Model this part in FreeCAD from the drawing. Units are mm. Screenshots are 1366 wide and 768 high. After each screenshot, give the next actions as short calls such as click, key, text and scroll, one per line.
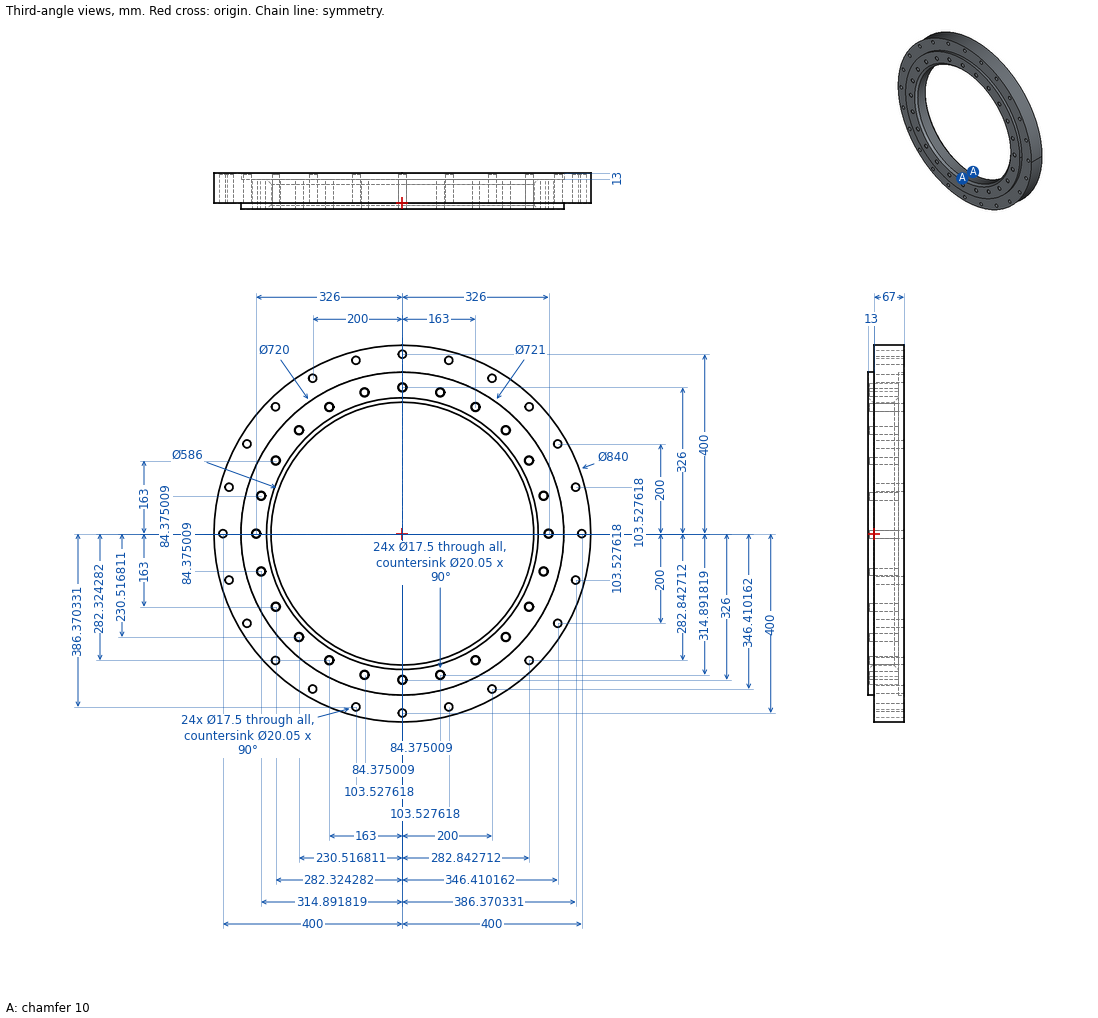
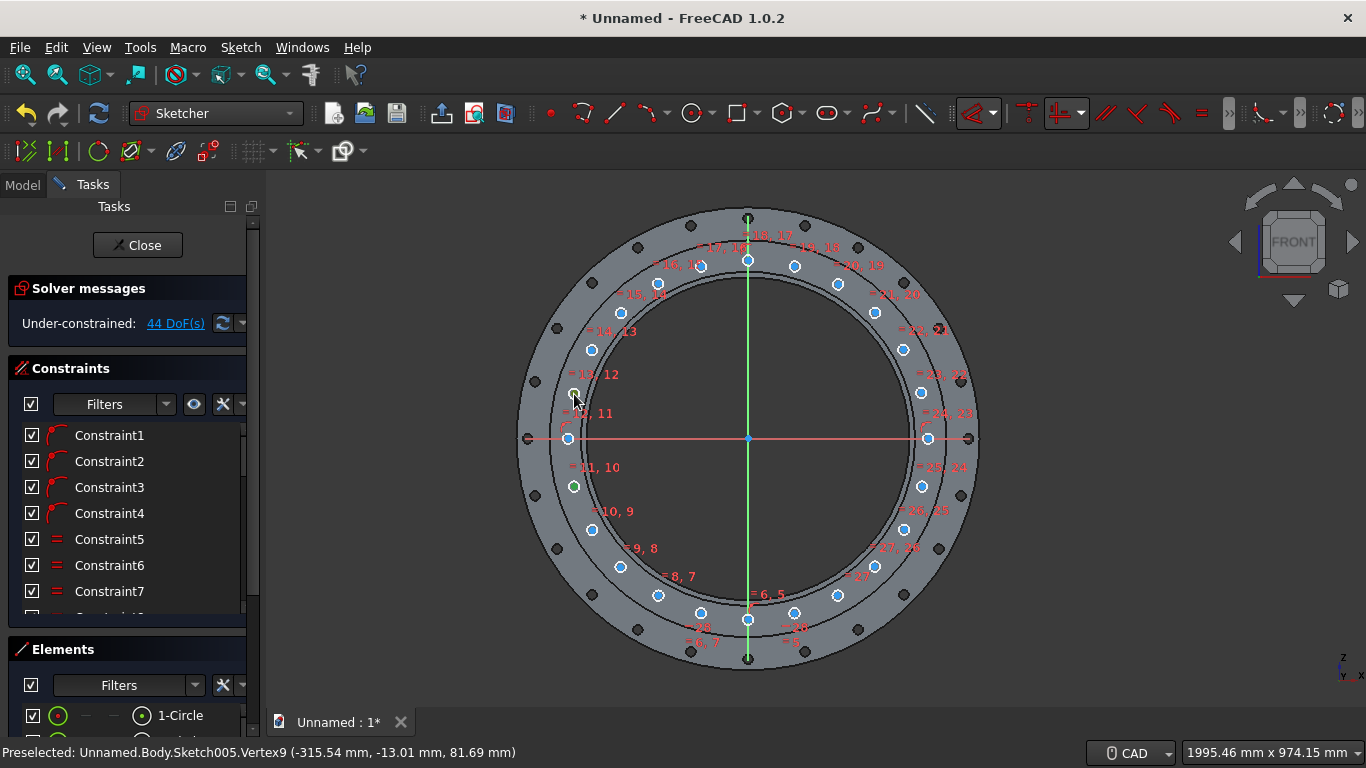
click(1084, 114)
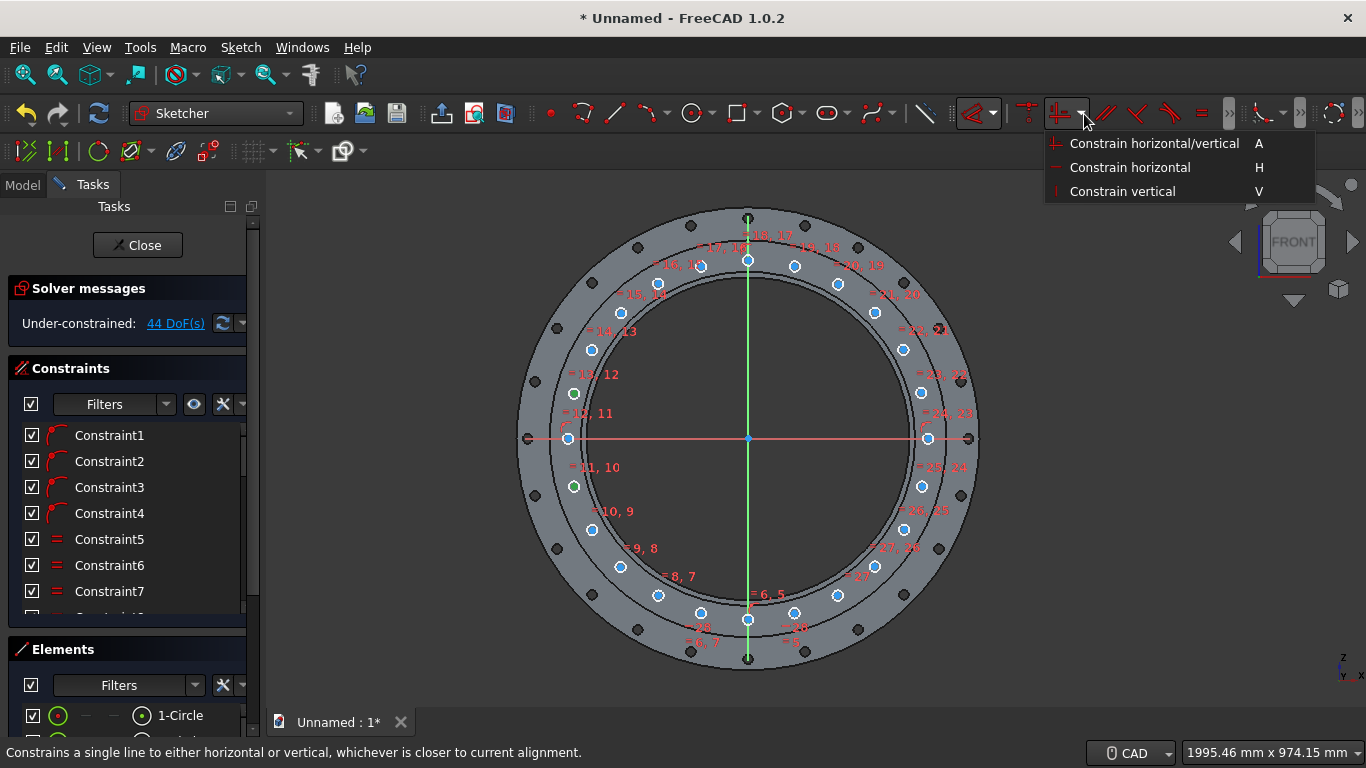
click(1180, 191)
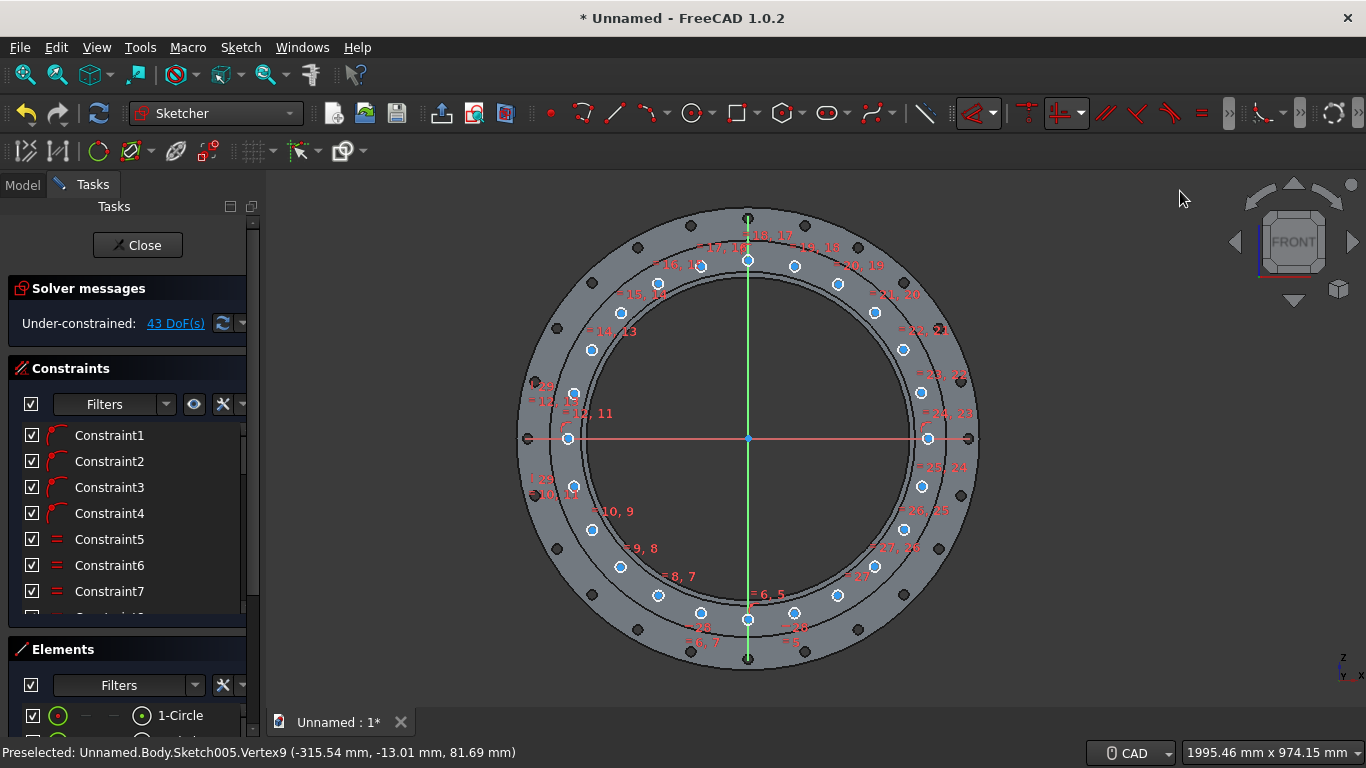
click(592, 530)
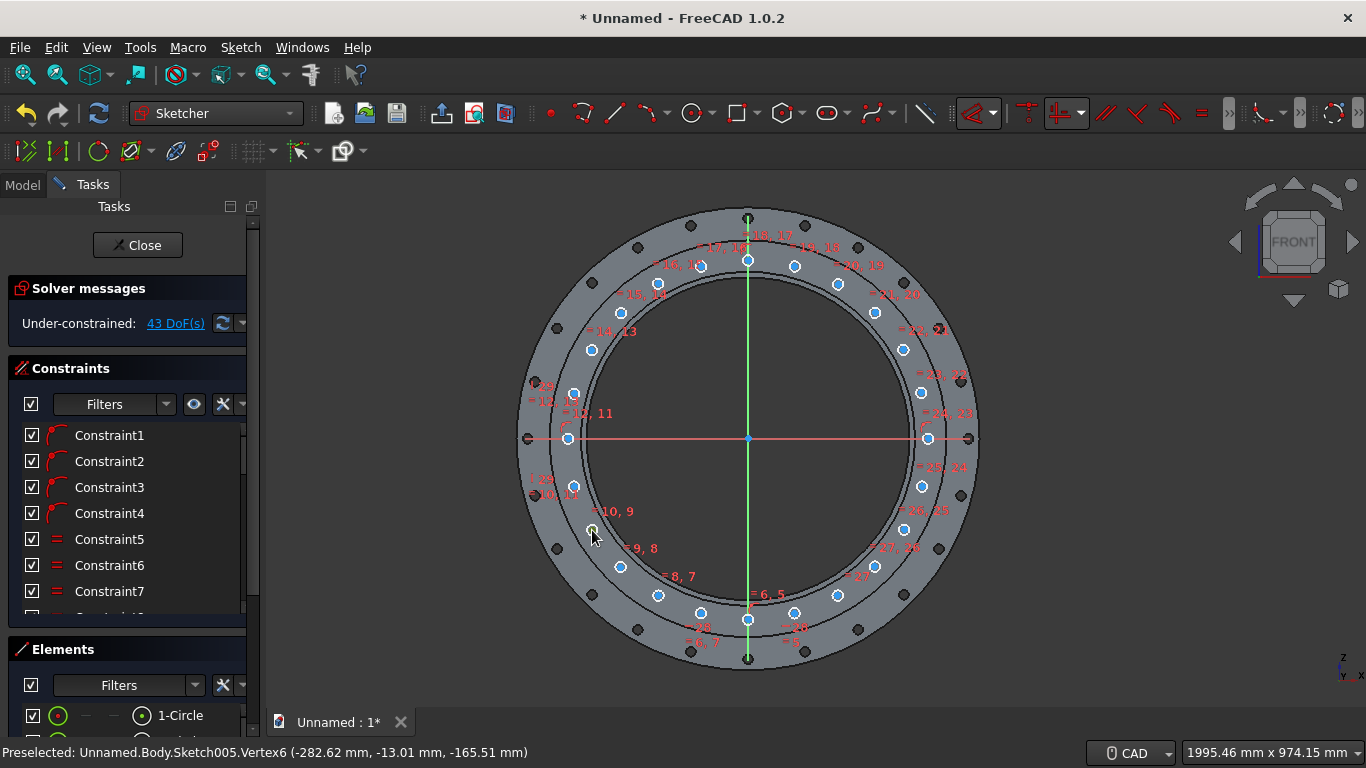
click(592, 350)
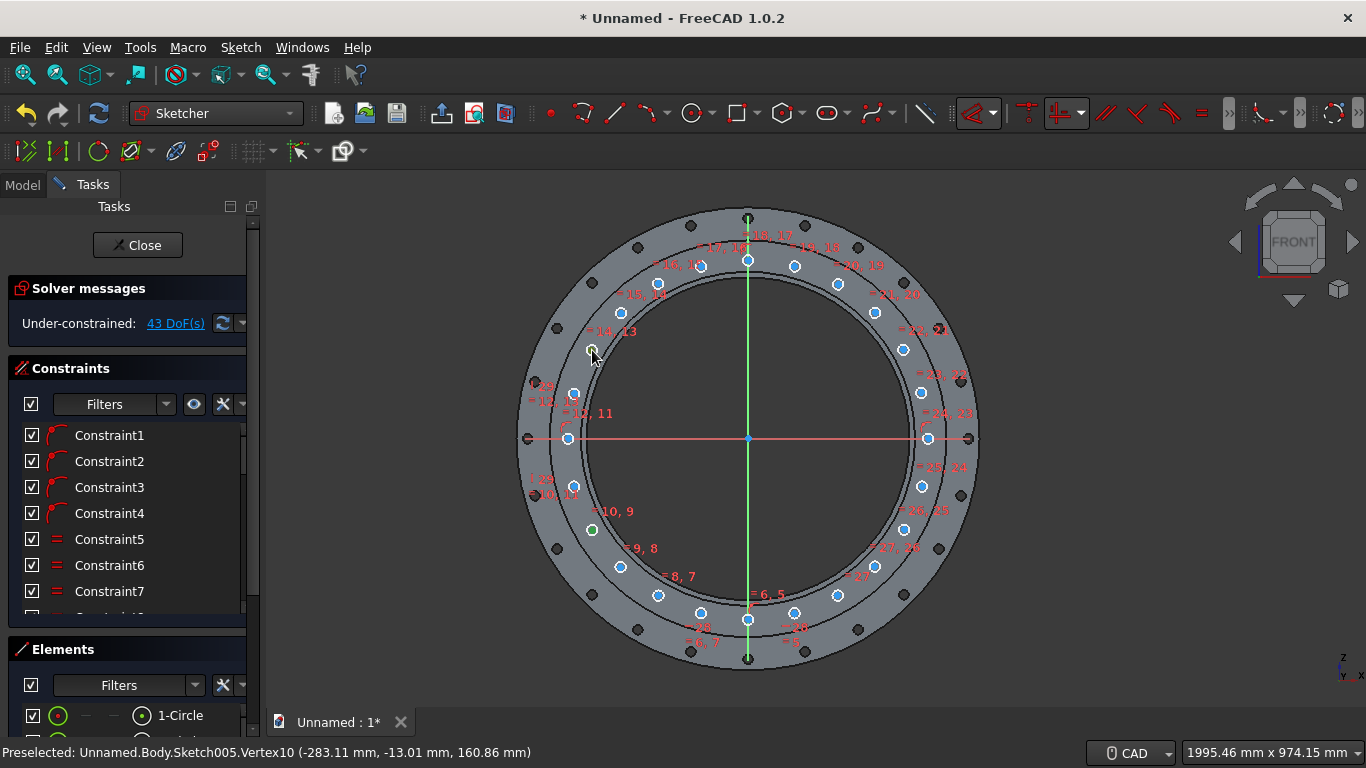
key(v)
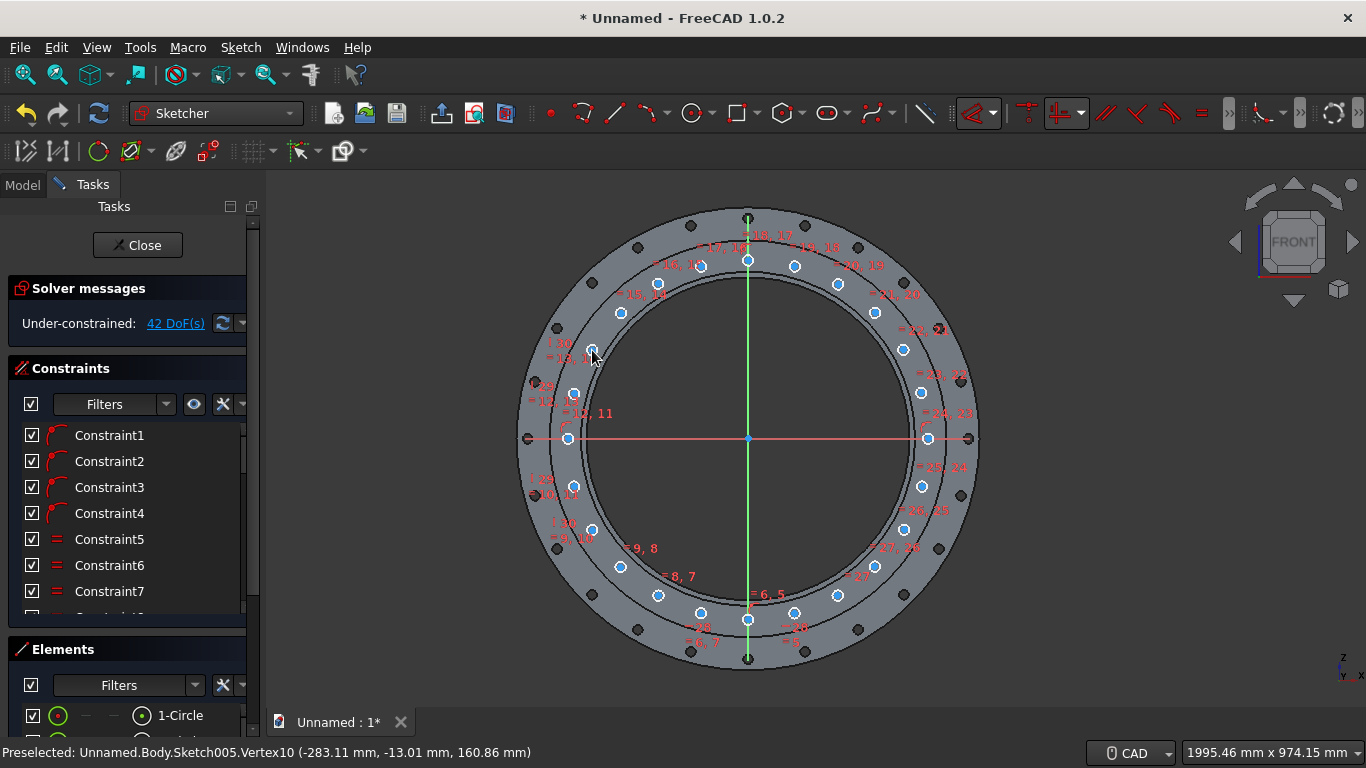
click(621, 567)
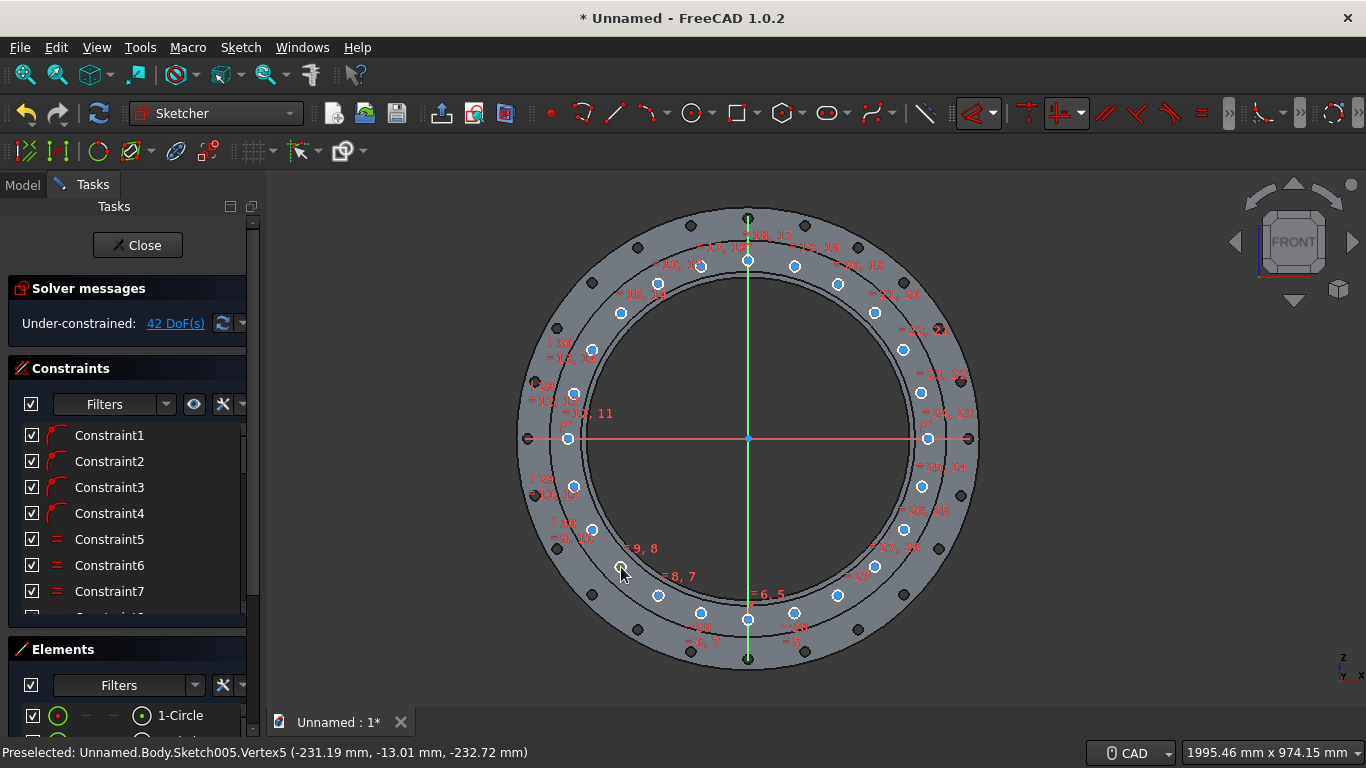
click(621, 313)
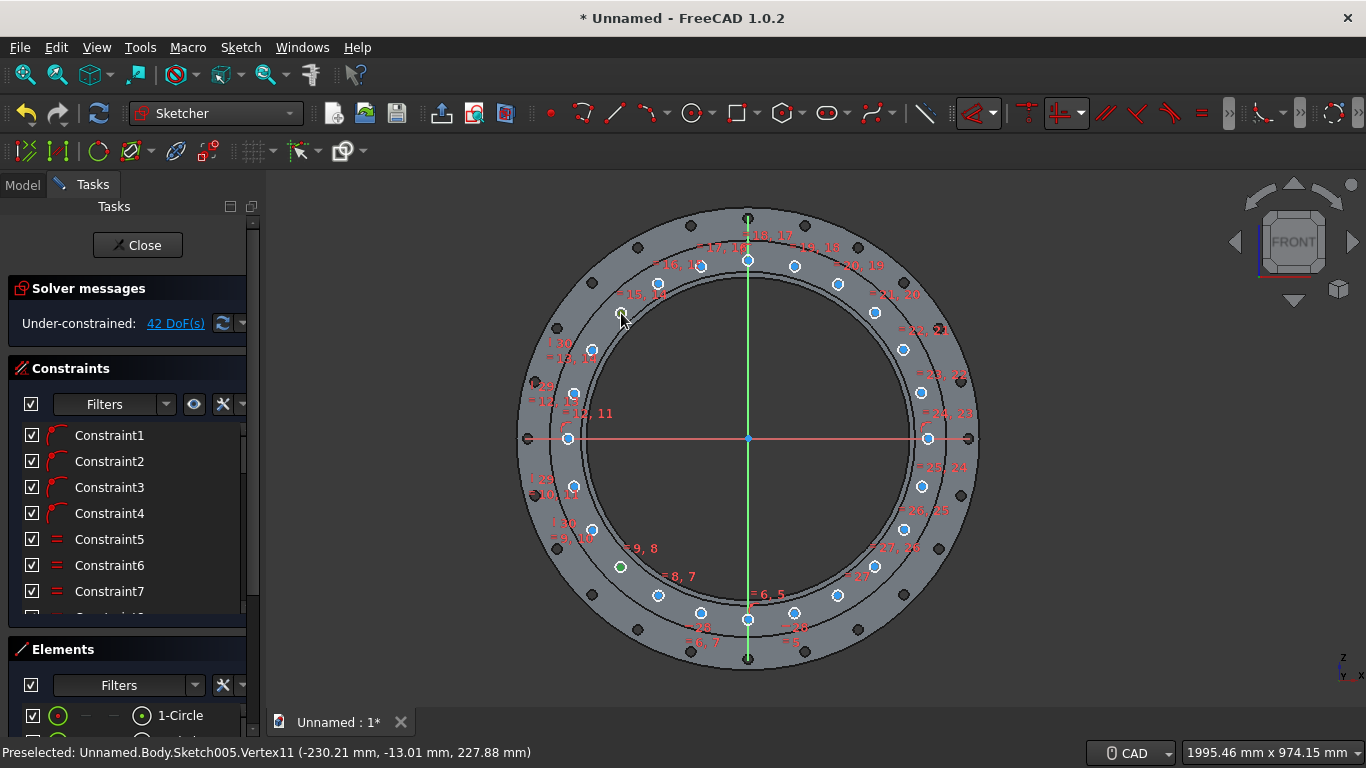
key(v)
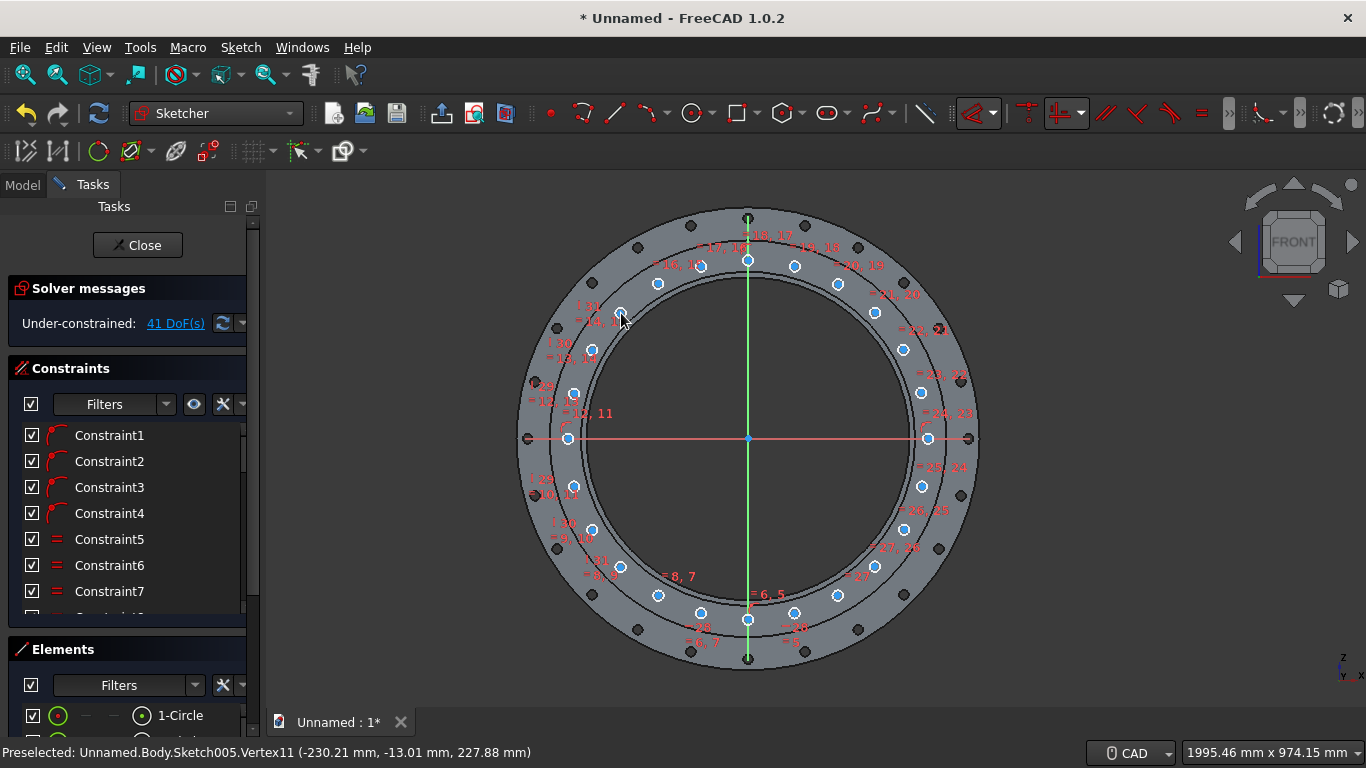
click(701, 267)